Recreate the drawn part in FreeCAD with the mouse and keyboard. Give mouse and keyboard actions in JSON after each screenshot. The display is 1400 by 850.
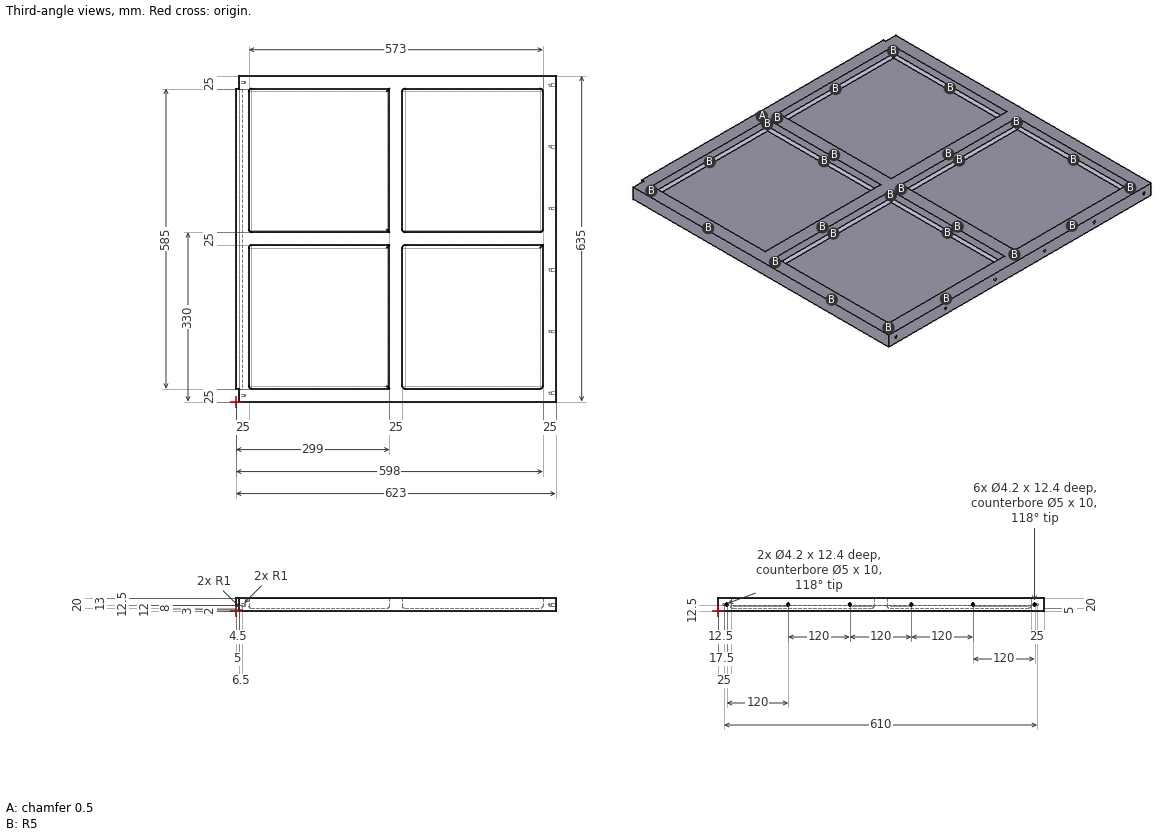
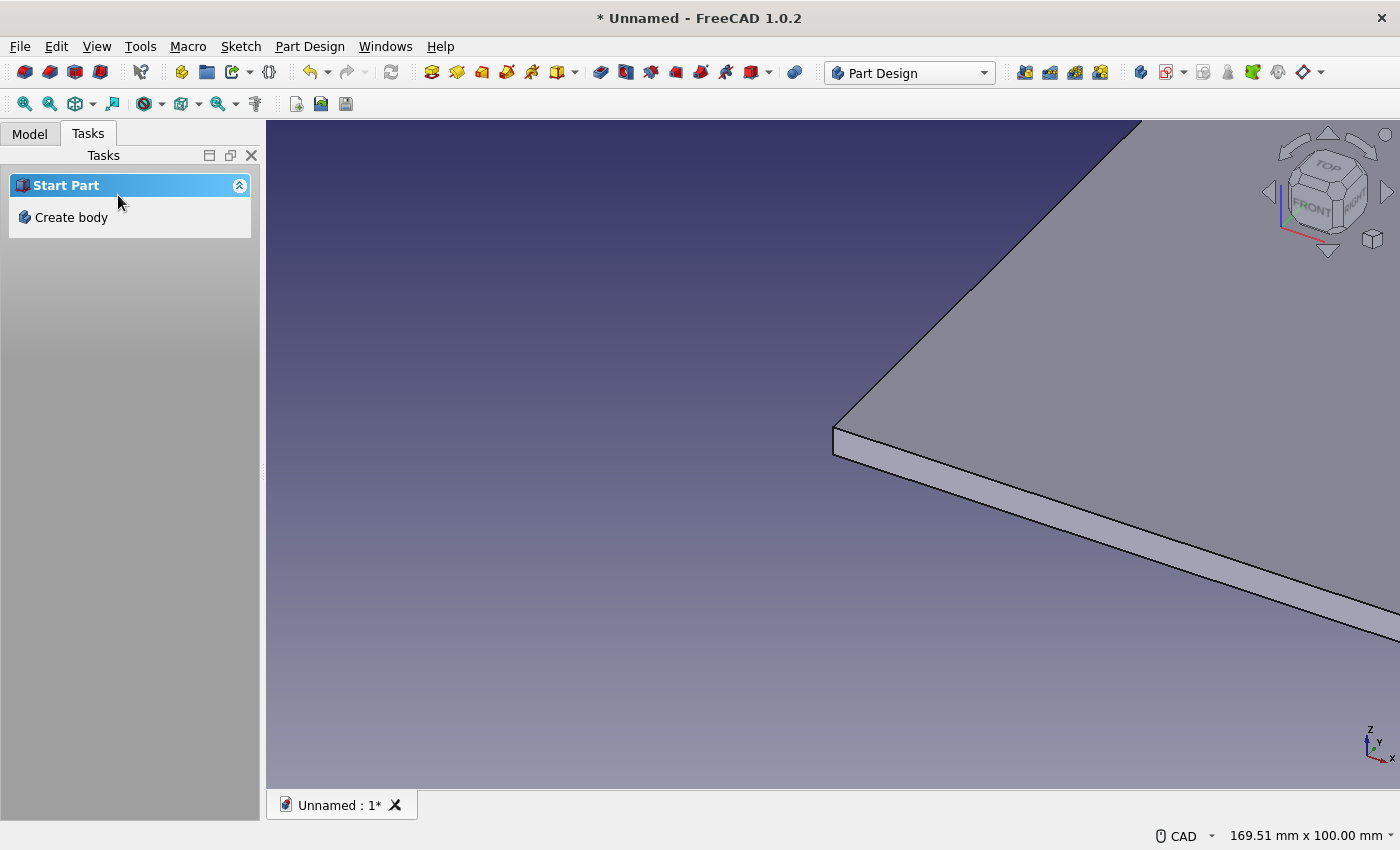
{"action": "left_click", "coordinate": [25, 104]}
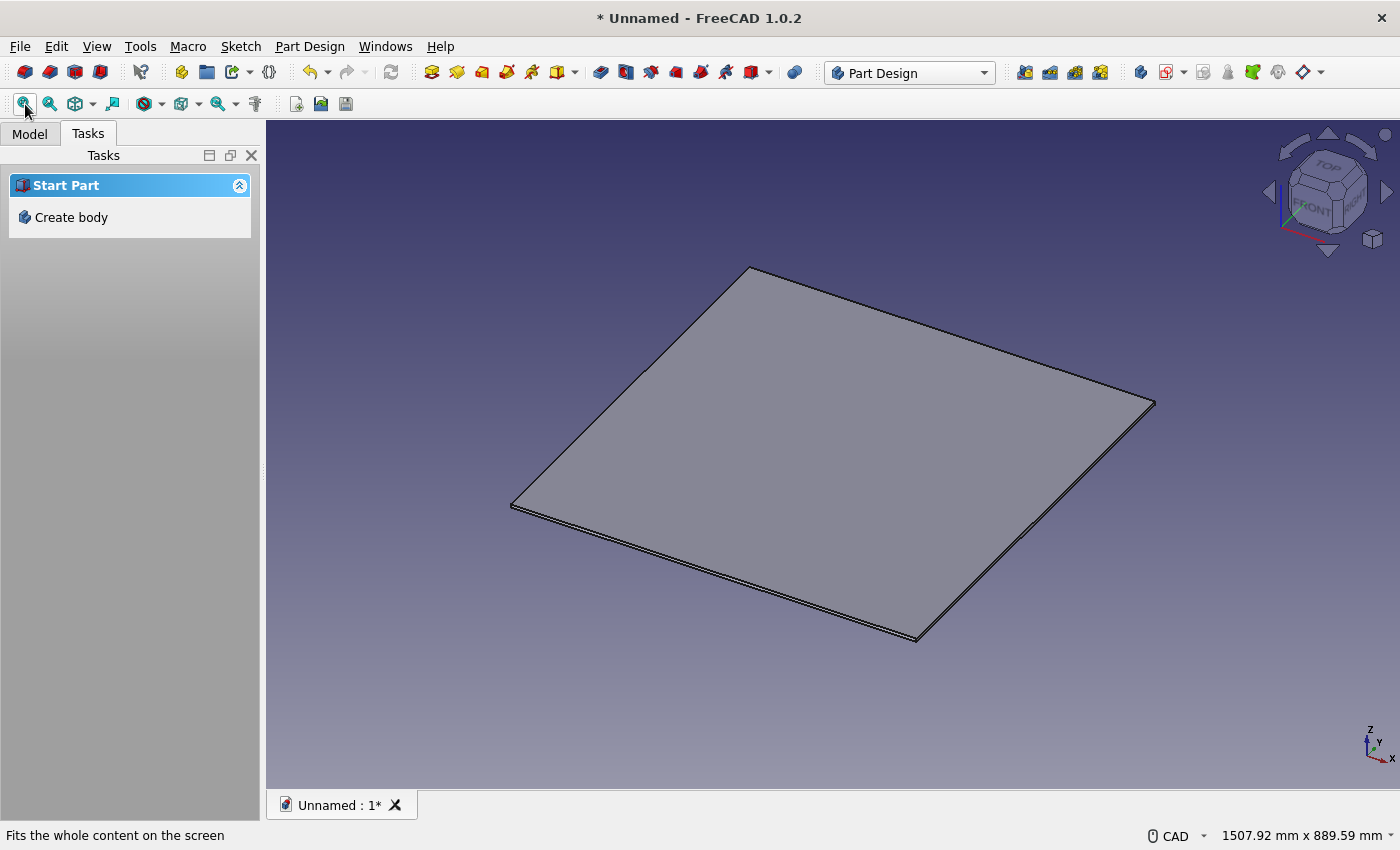
{"action": "left_click", "coordinate": [833, 452]}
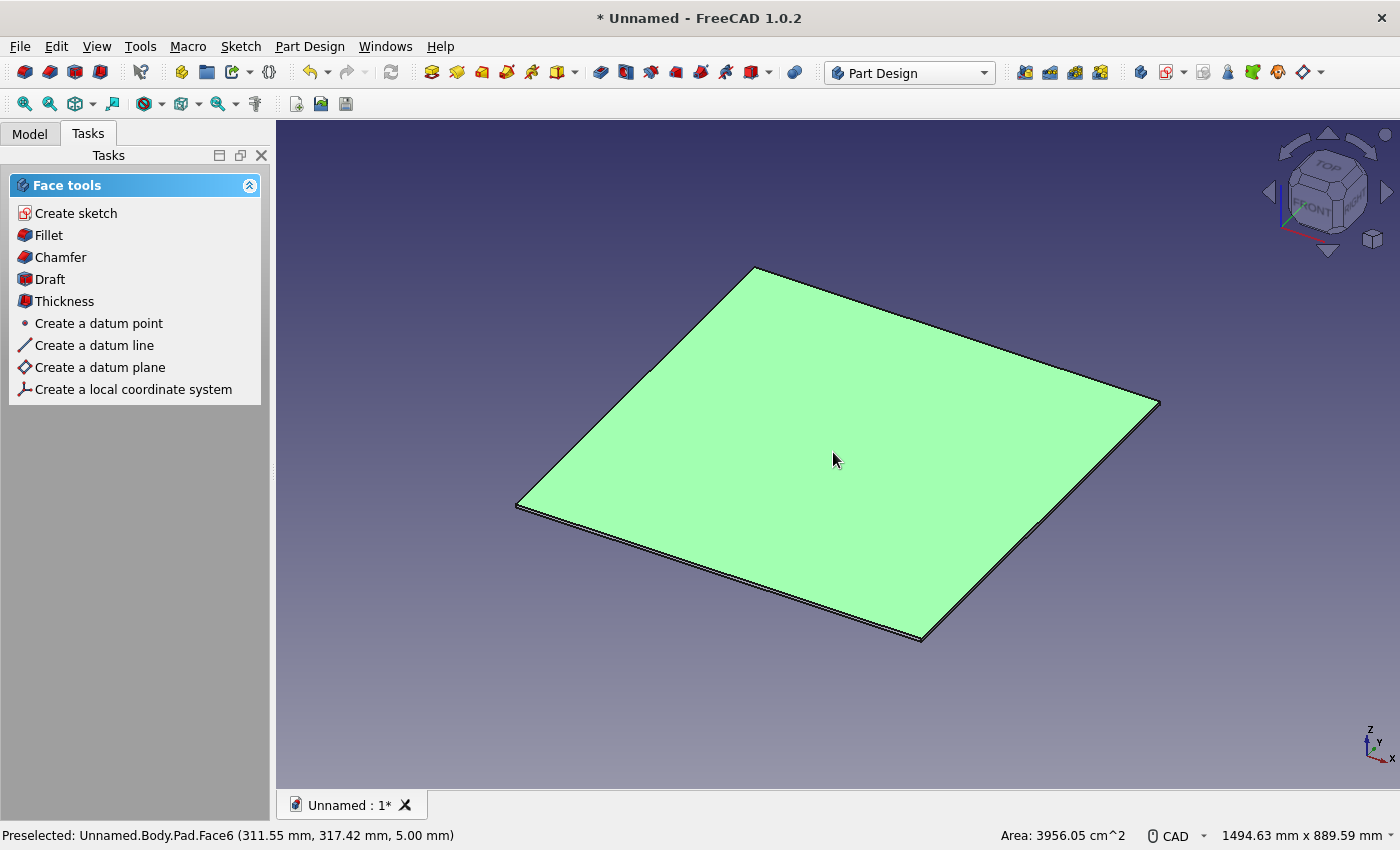
{"action": "left_click", "coordinate": [1166, 72]}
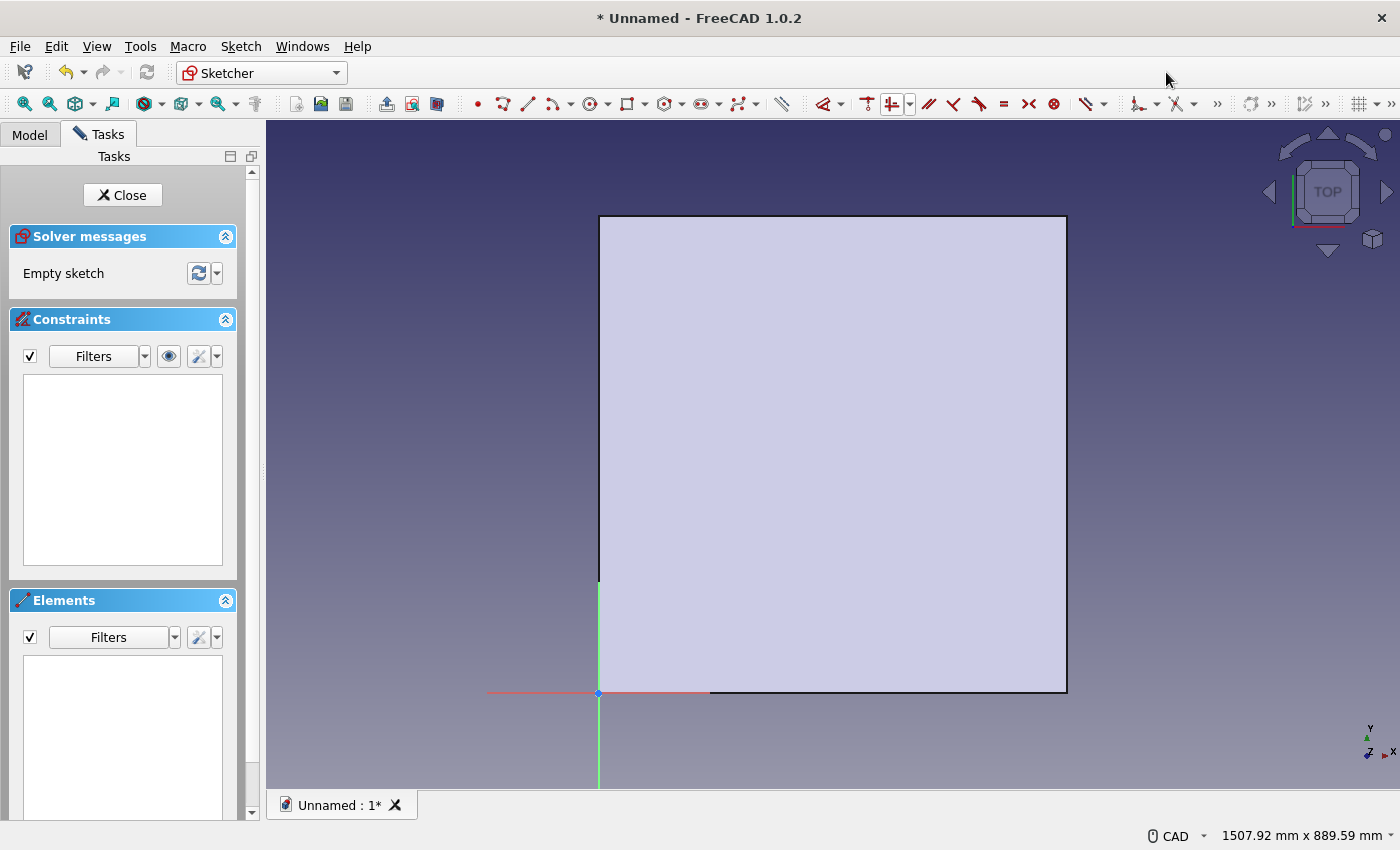
{"action": "key", "text": "g r"}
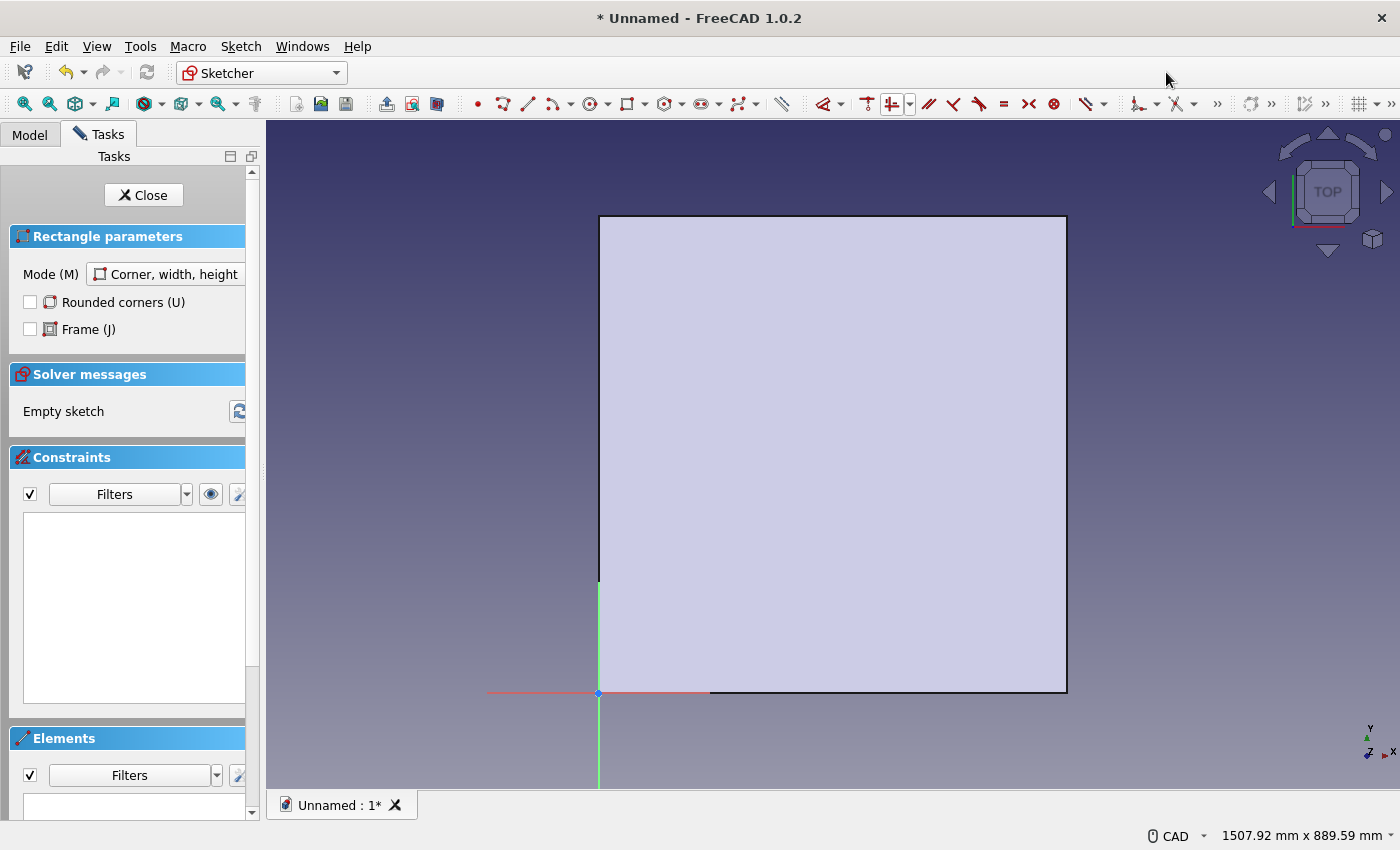
{"action": "left_click", "coordinate": [599, 693]}
{"action": "left_click", "coordinate": [618, 216]}
{"action": "key", "text": "Escape"}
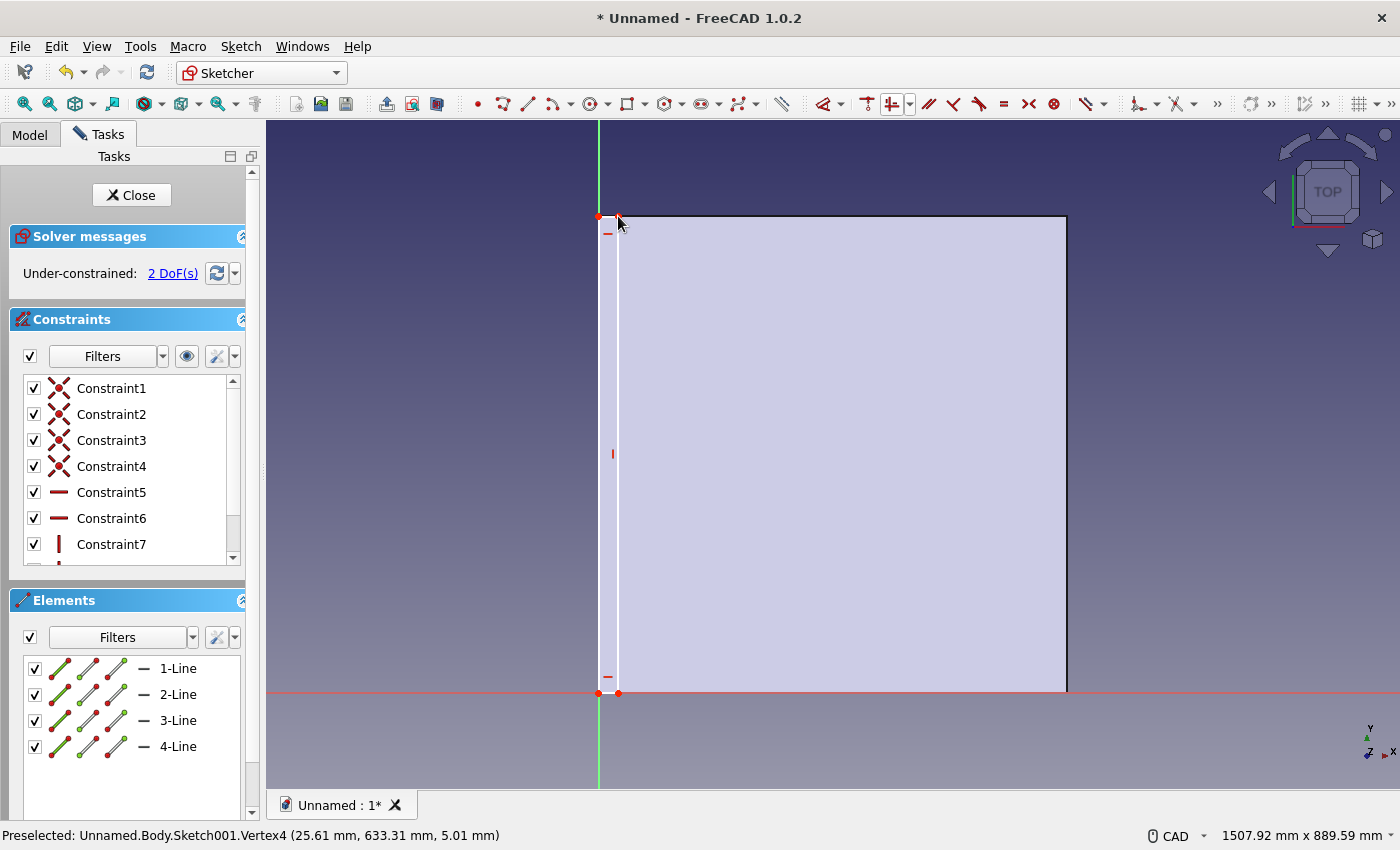
{"action": "left_click", "coordinate": [822, 104]}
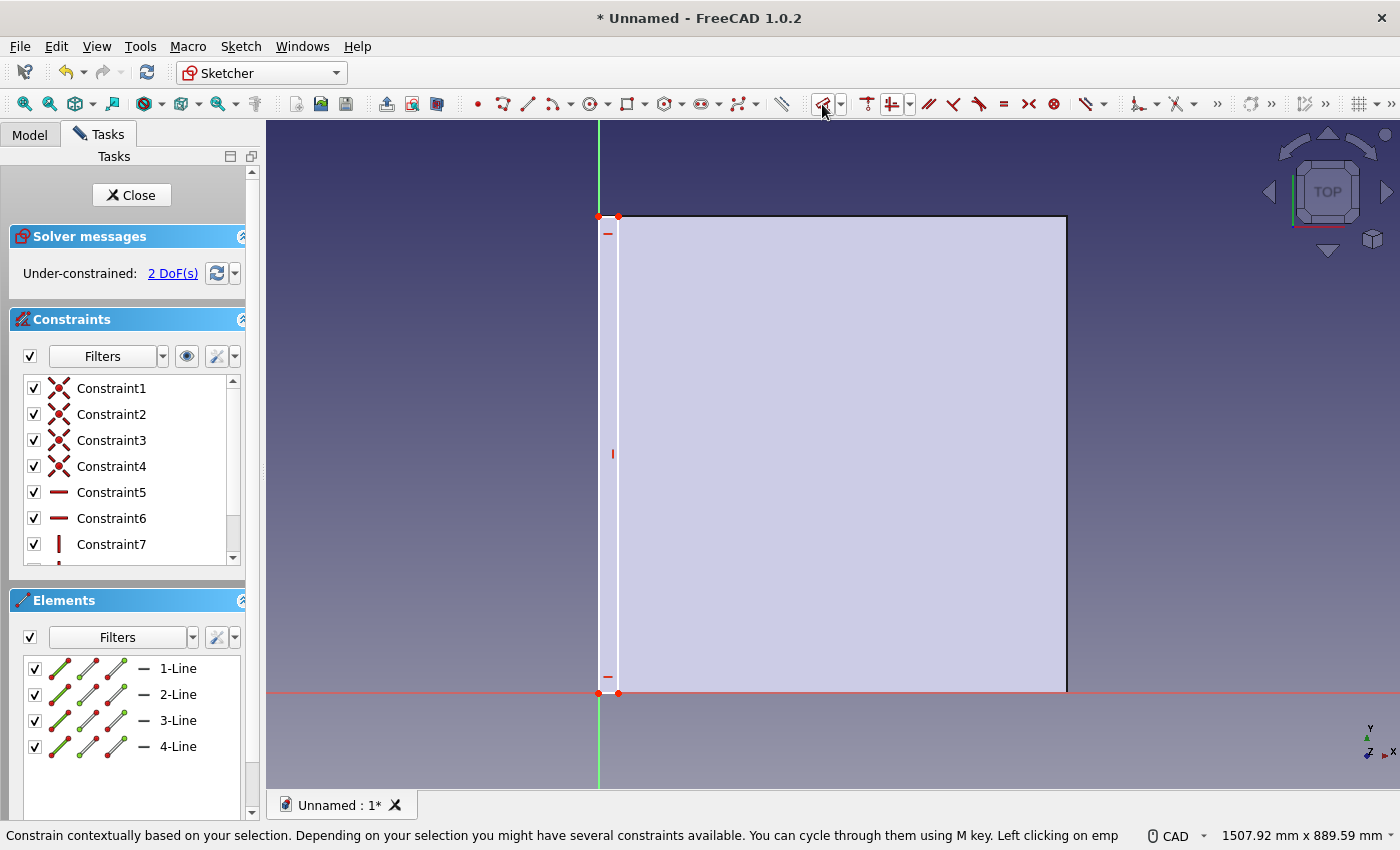
{"action": "scroll", "coordinate": [608, 693], "scroll_direction": "up", "scroll_amount": 4}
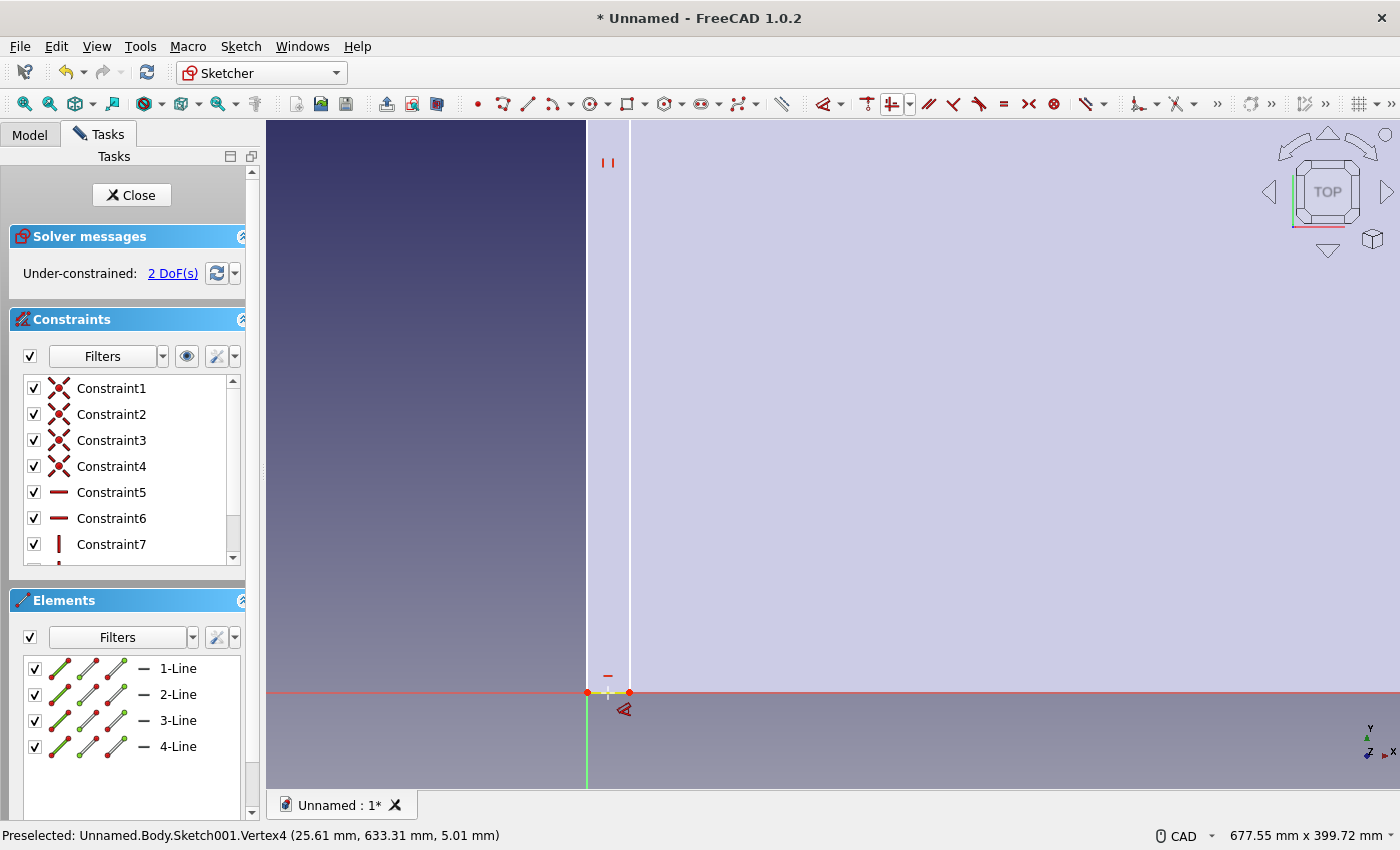
{"action": "left_click", "coordinate": [608, 693]}
{"action": "left_click", "coordinate": [608, 727]}